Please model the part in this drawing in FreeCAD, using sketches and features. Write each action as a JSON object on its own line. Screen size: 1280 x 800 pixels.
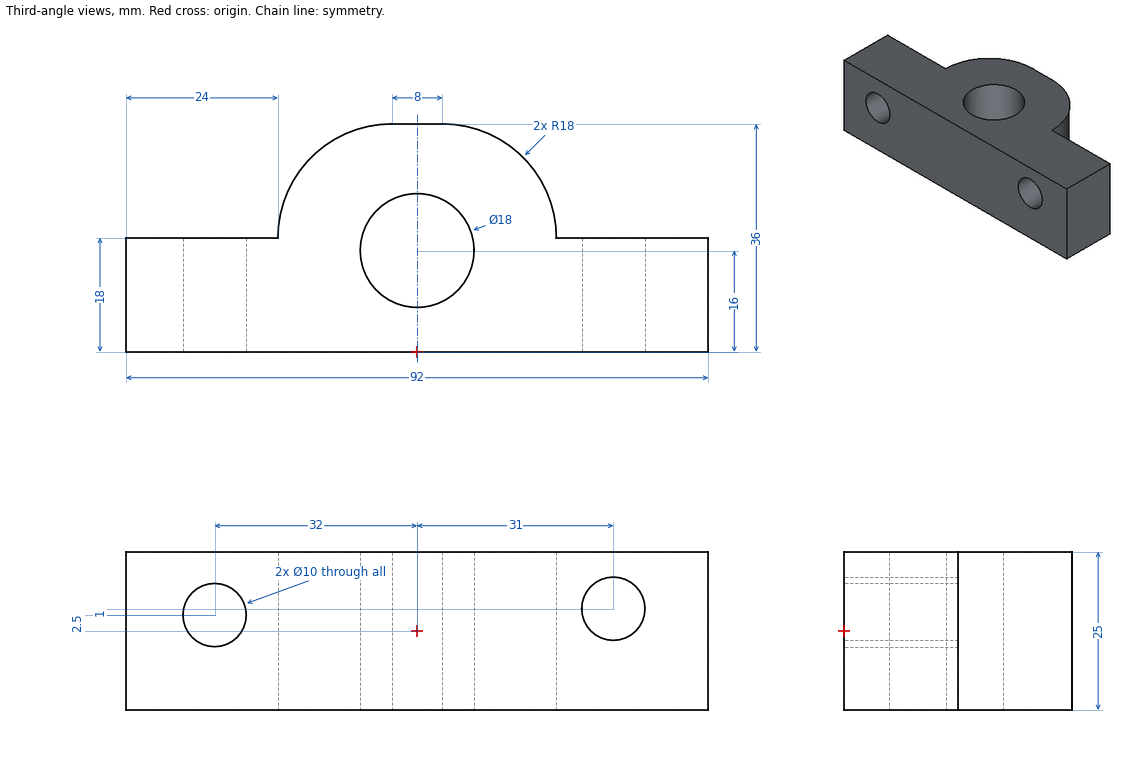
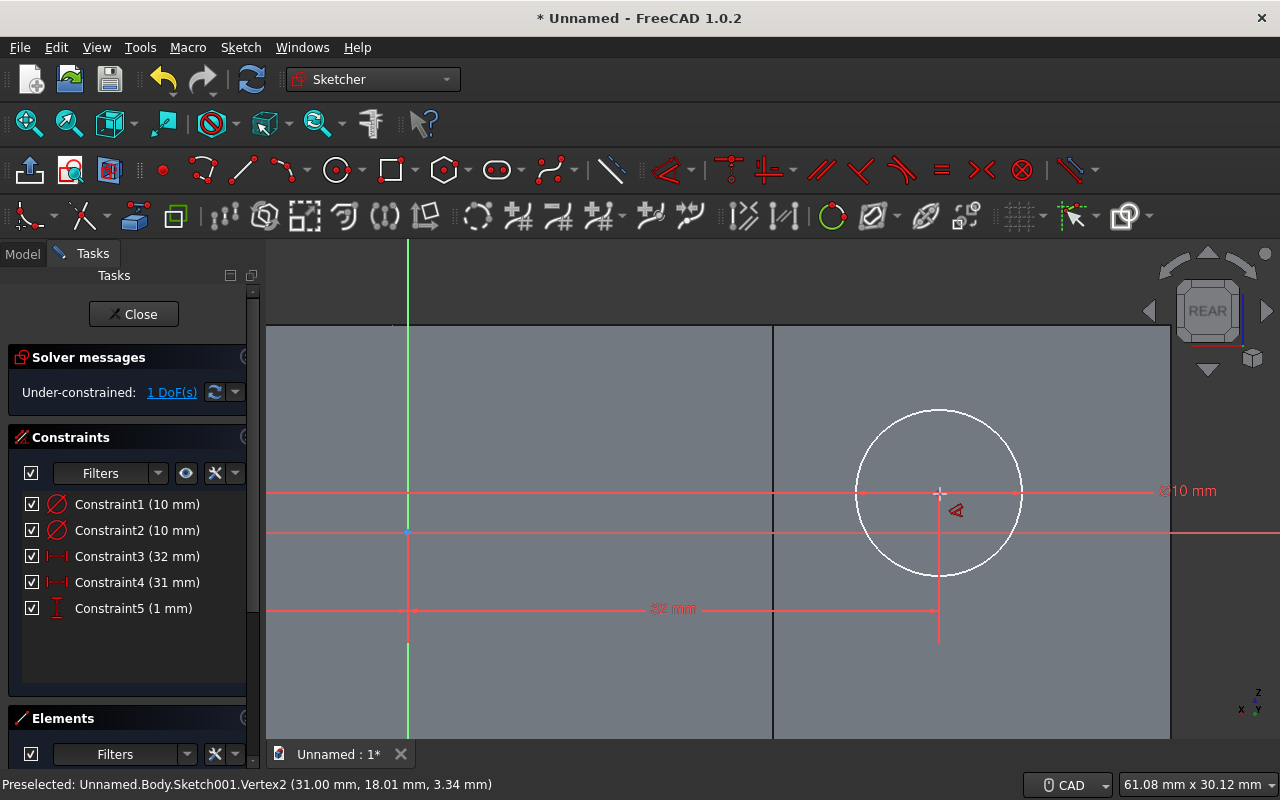
{"action": "left_click", "coordinate": [939, 493]}
{"action": "left_click", "coordinate": [973, 513]}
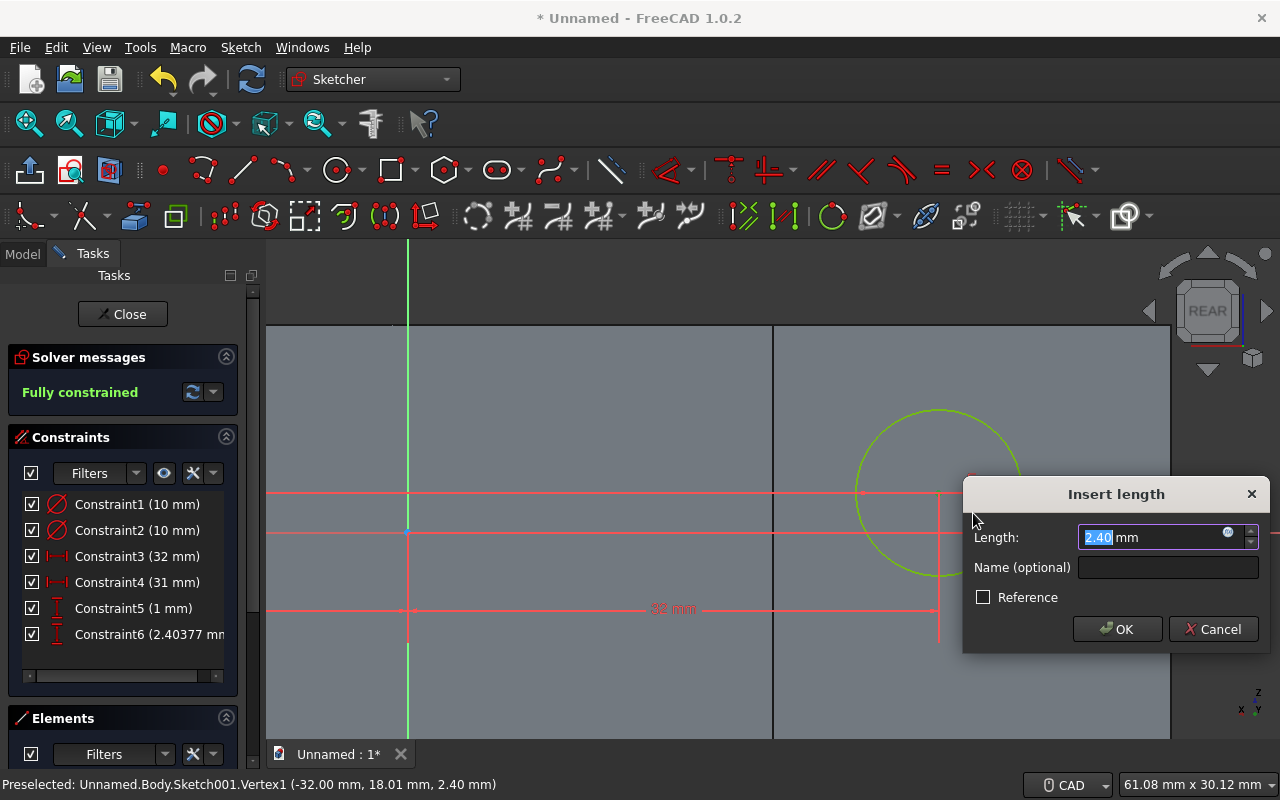
{"action": "type", "text": "2.5"}
{"action": "key", "text": "Return"}
{"action": "key", "text": "Escape"}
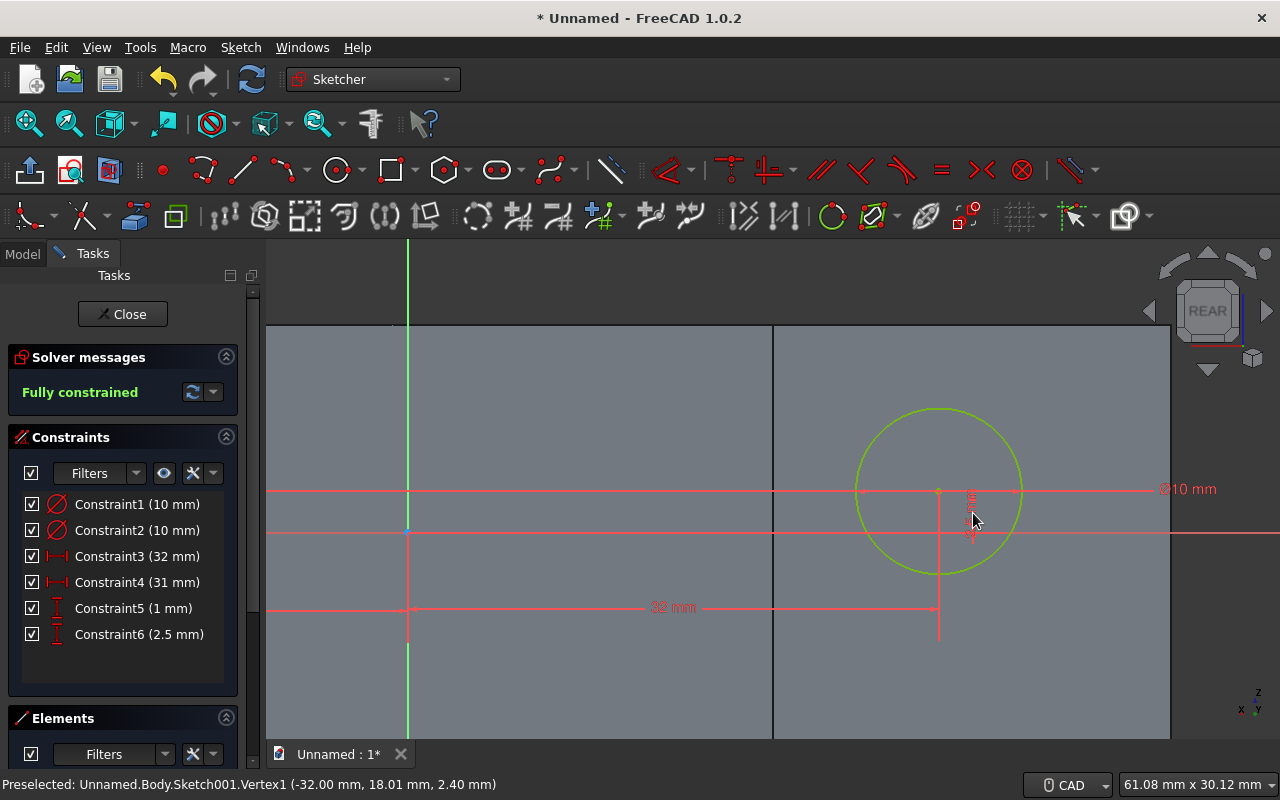
{"action": "left_click", "coordinate": [123, 314]}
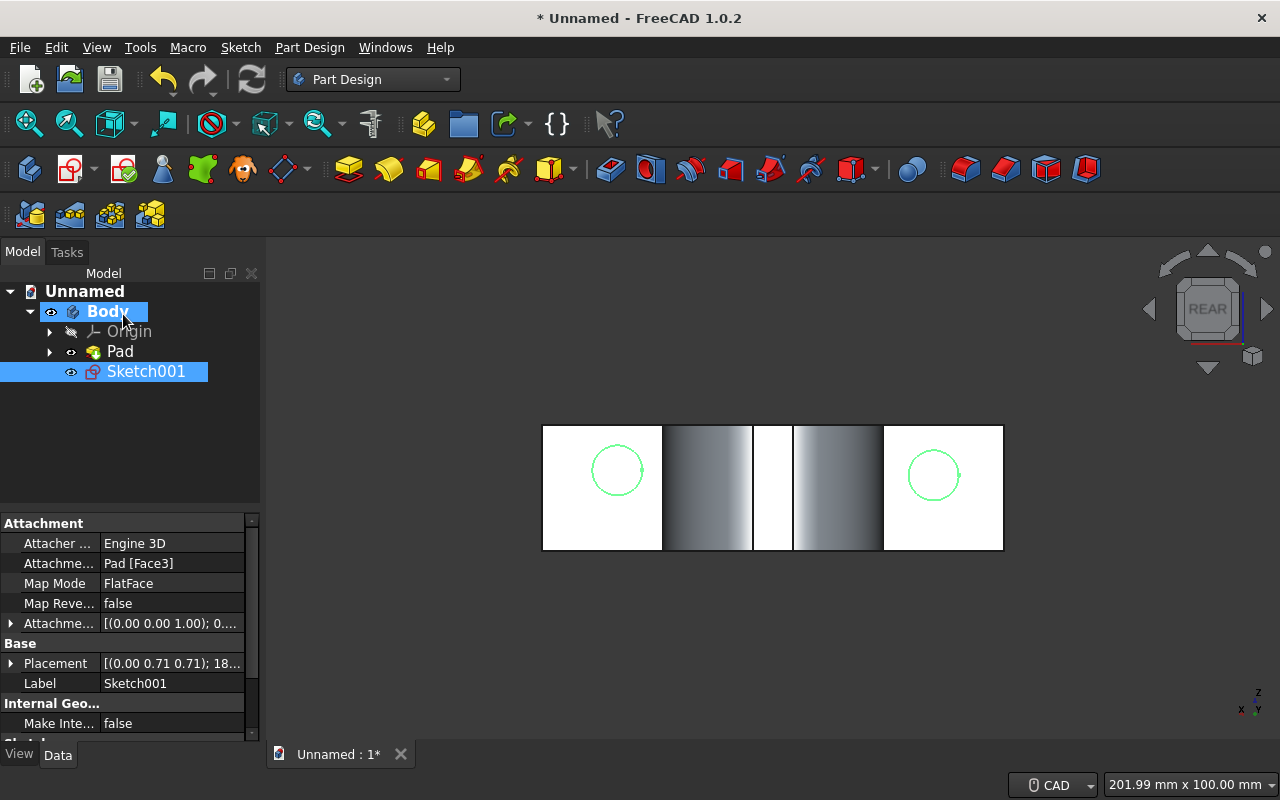
{"action": "left_click", "coordinate": [652, 170]}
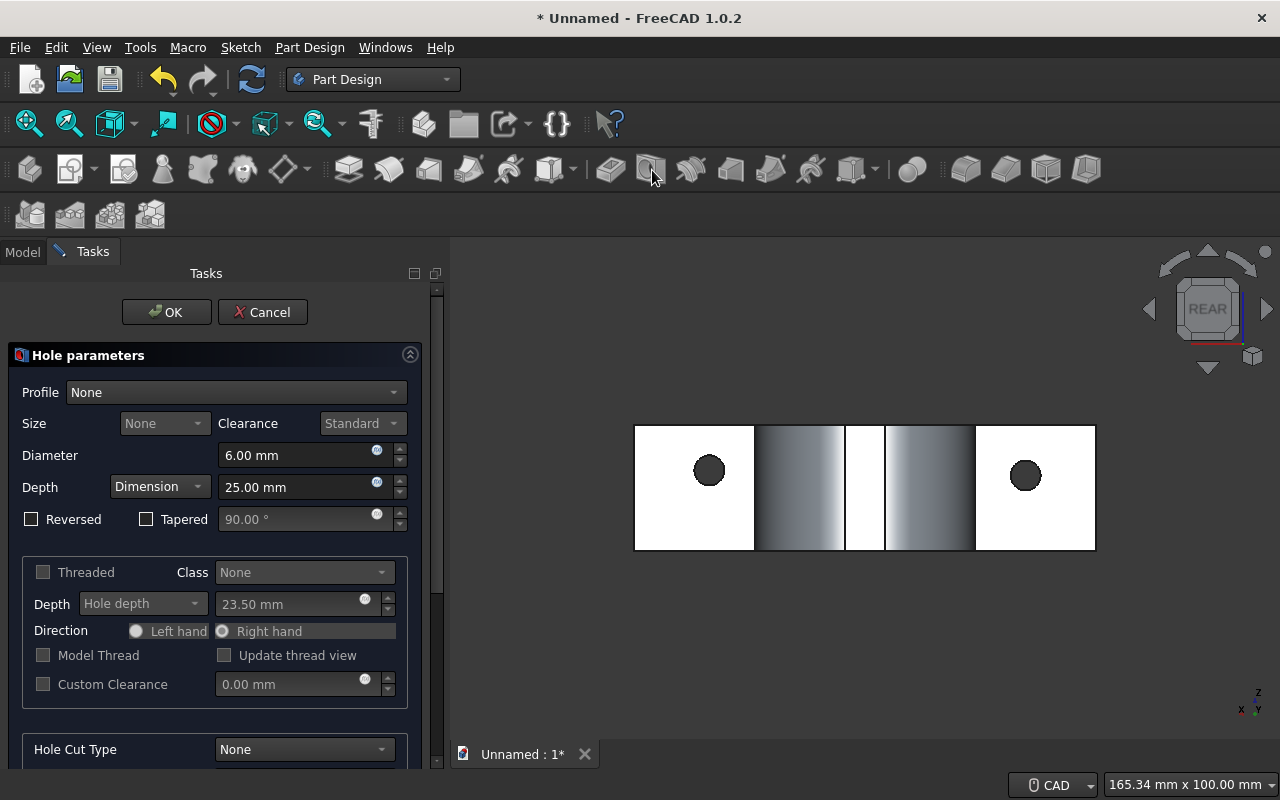
{"action": "triple_click", "coordinate": [305, 455]}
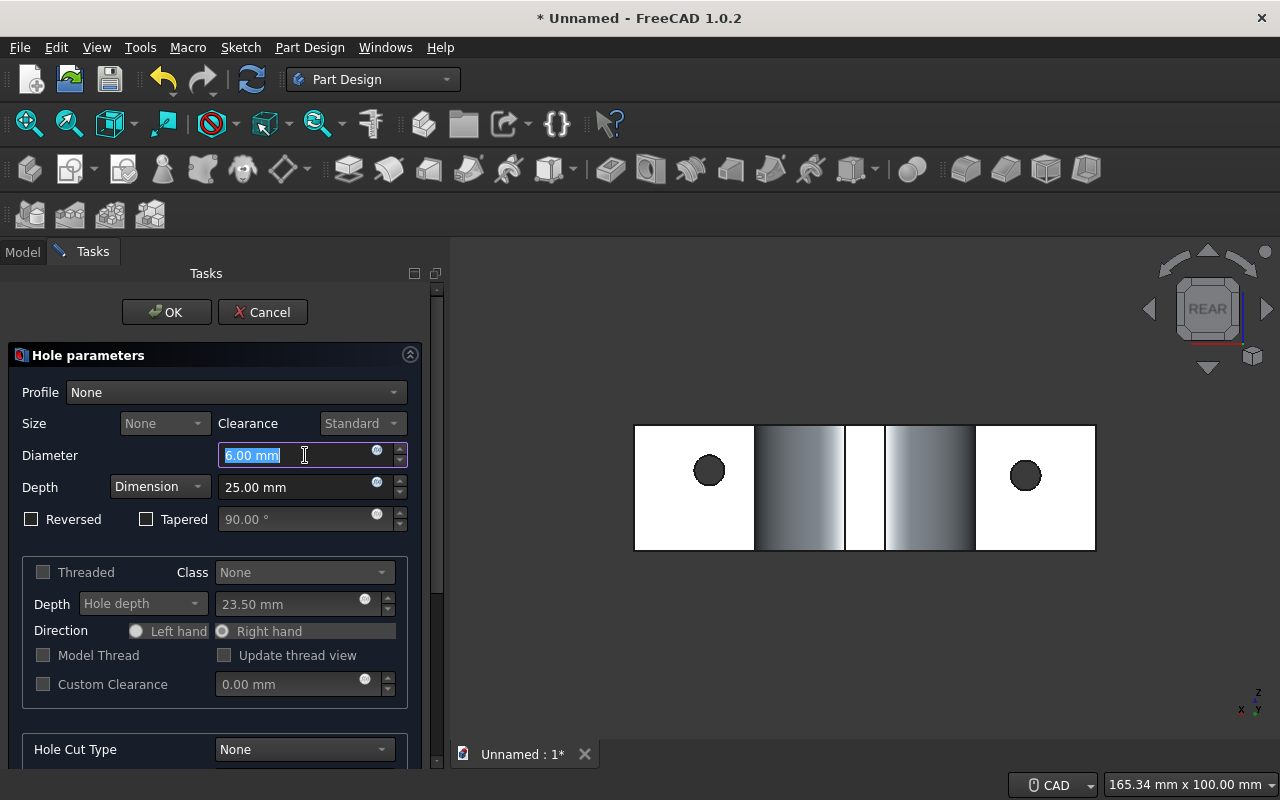
{"action": "type", "text": "10"}
{"action": "key", "text": "Tab"}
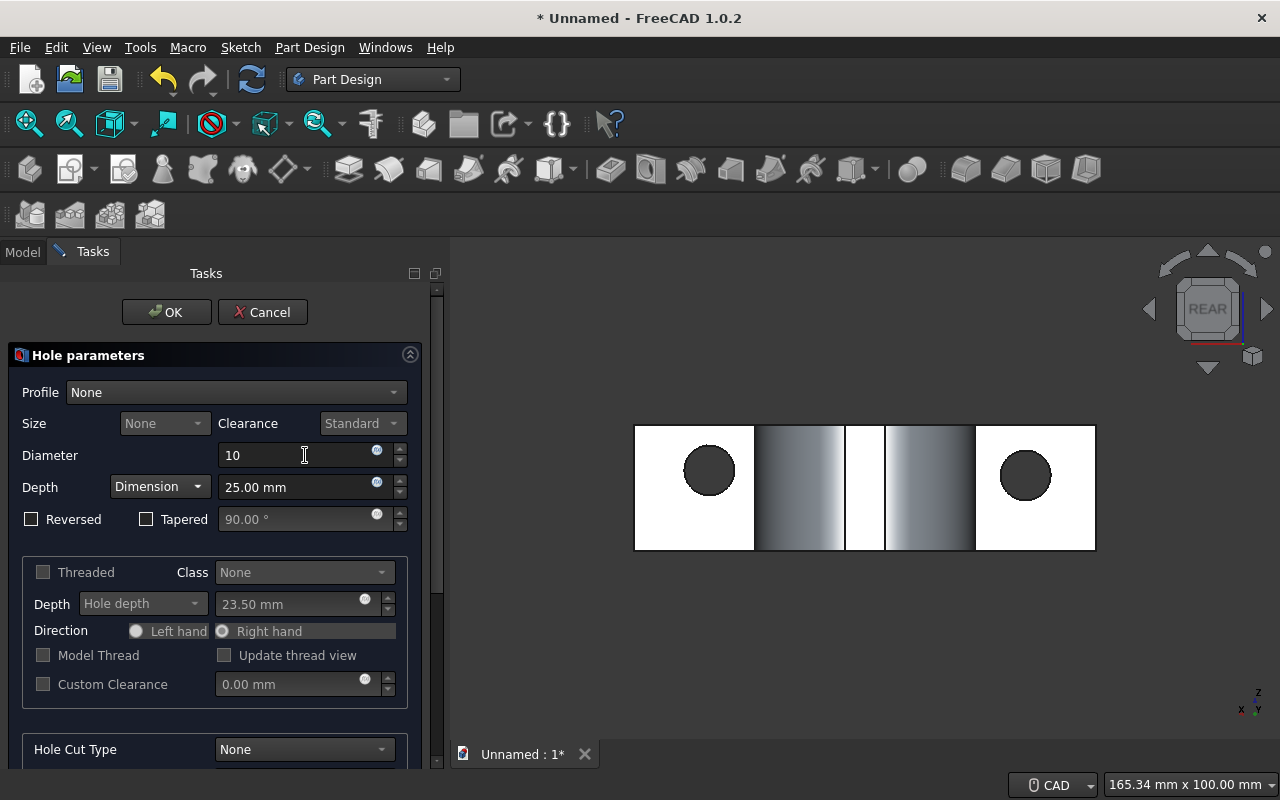
{"action": "left_click", "coordinate": [161, 486]}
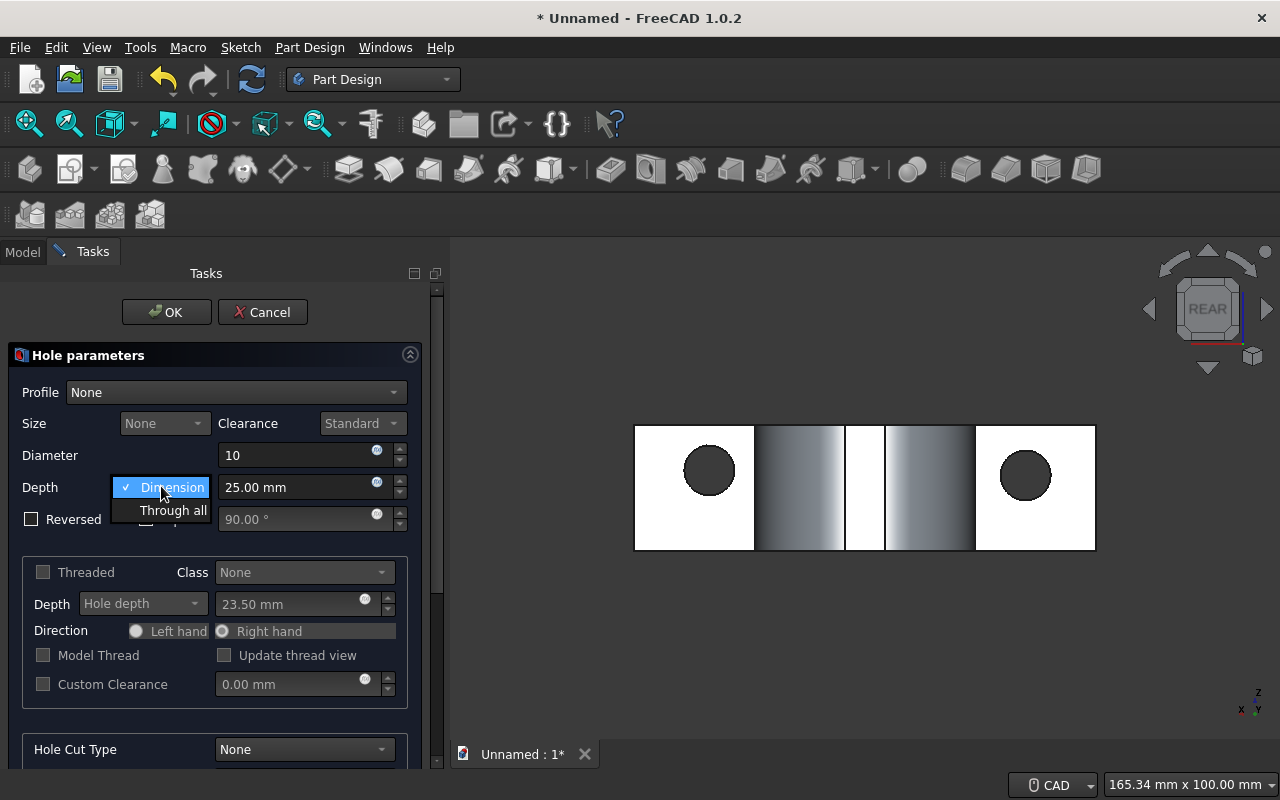
{"action": "left_click", "coordinate": [160, 510]}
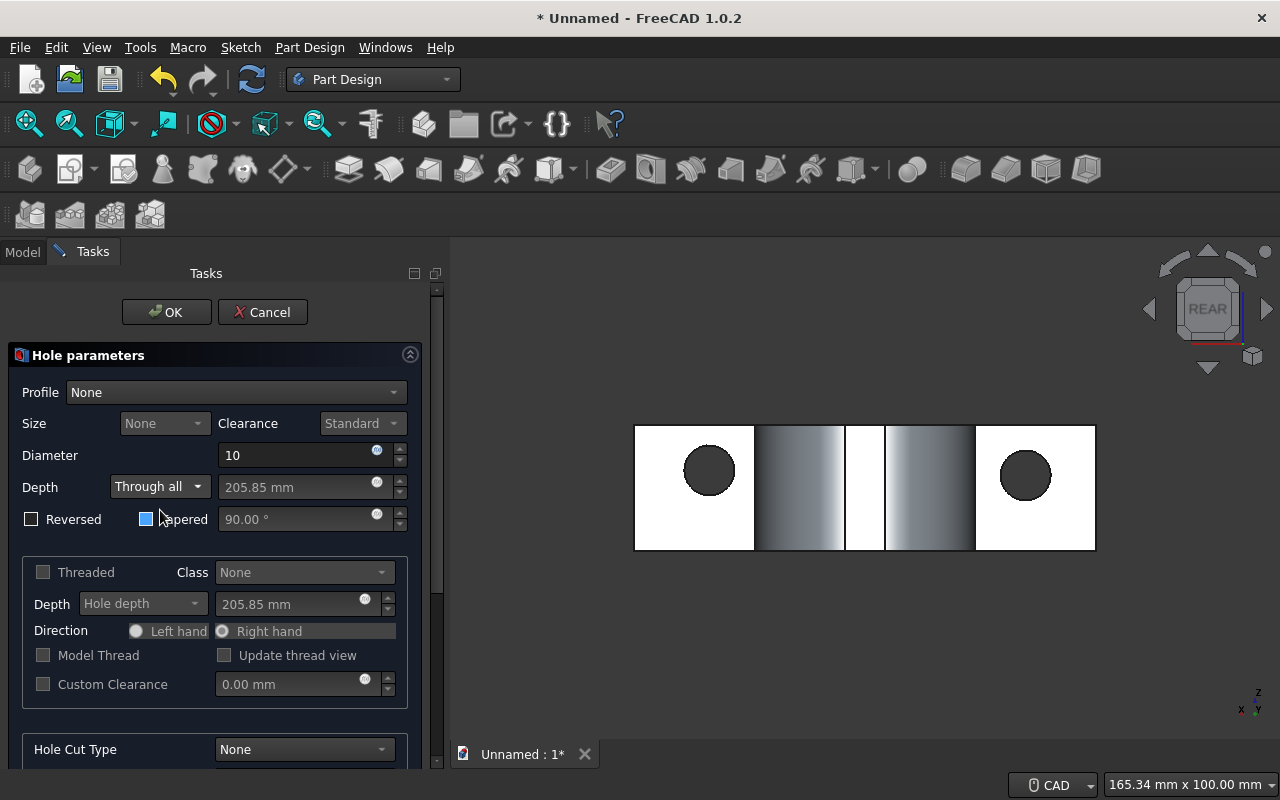
{"action": "left_click", "coordinate": [167, 312]}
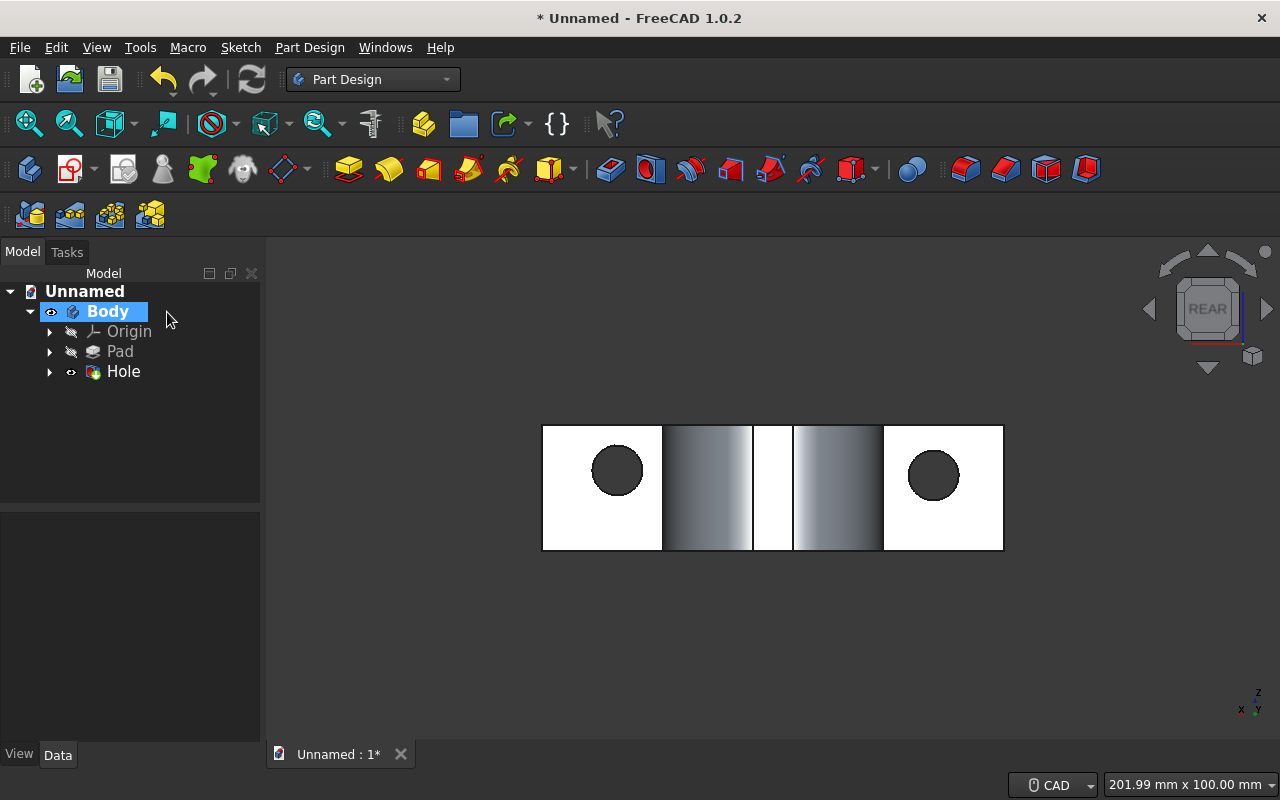
{"action": "key", "text": "0"}